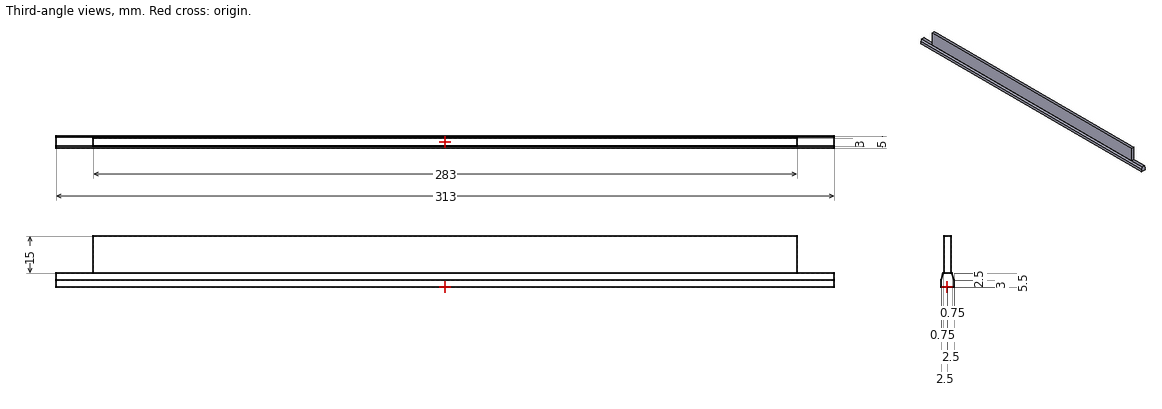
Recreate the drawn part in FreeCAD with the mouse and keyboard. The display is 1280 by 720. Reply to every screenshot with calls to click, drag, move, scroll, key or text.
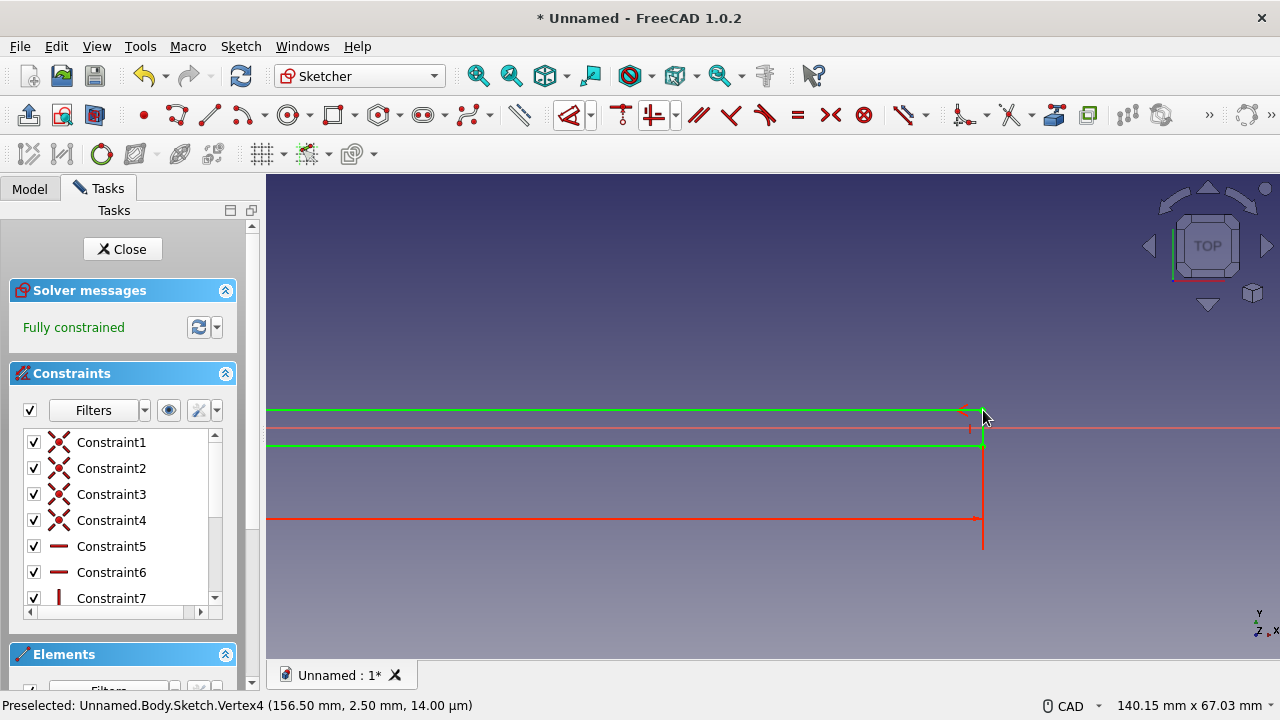
click(123, 249)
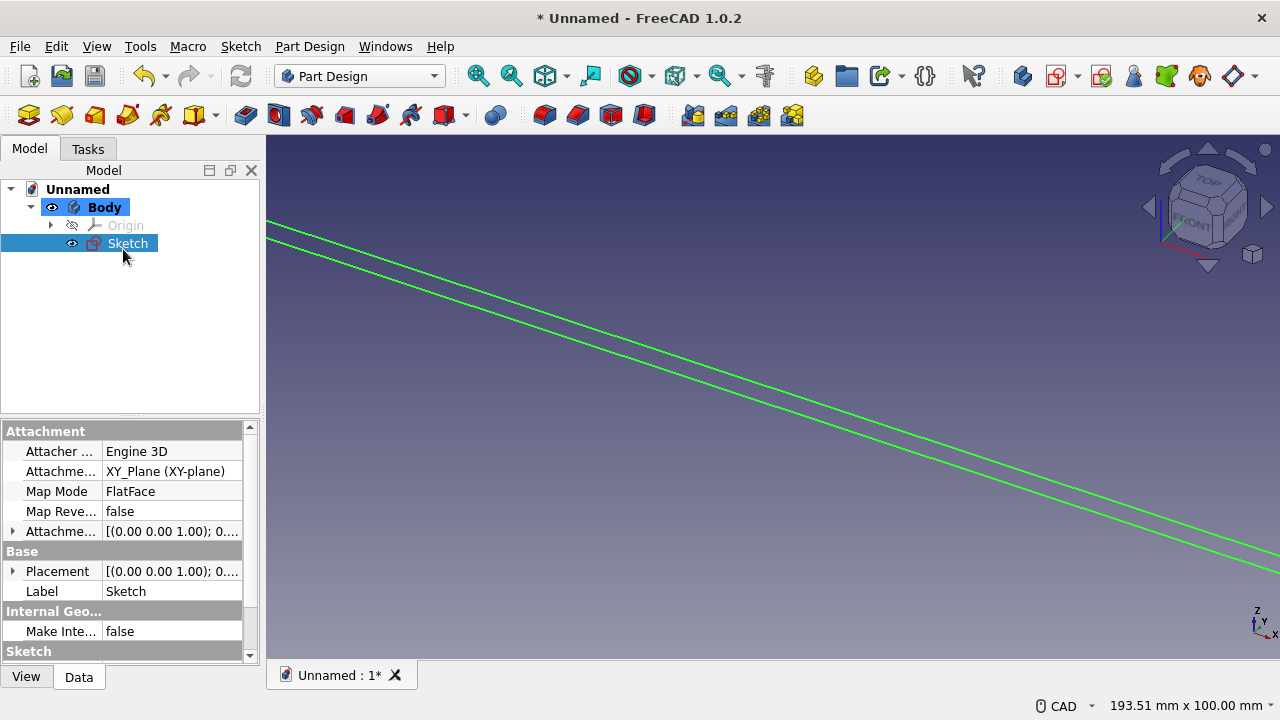
click(29, 116)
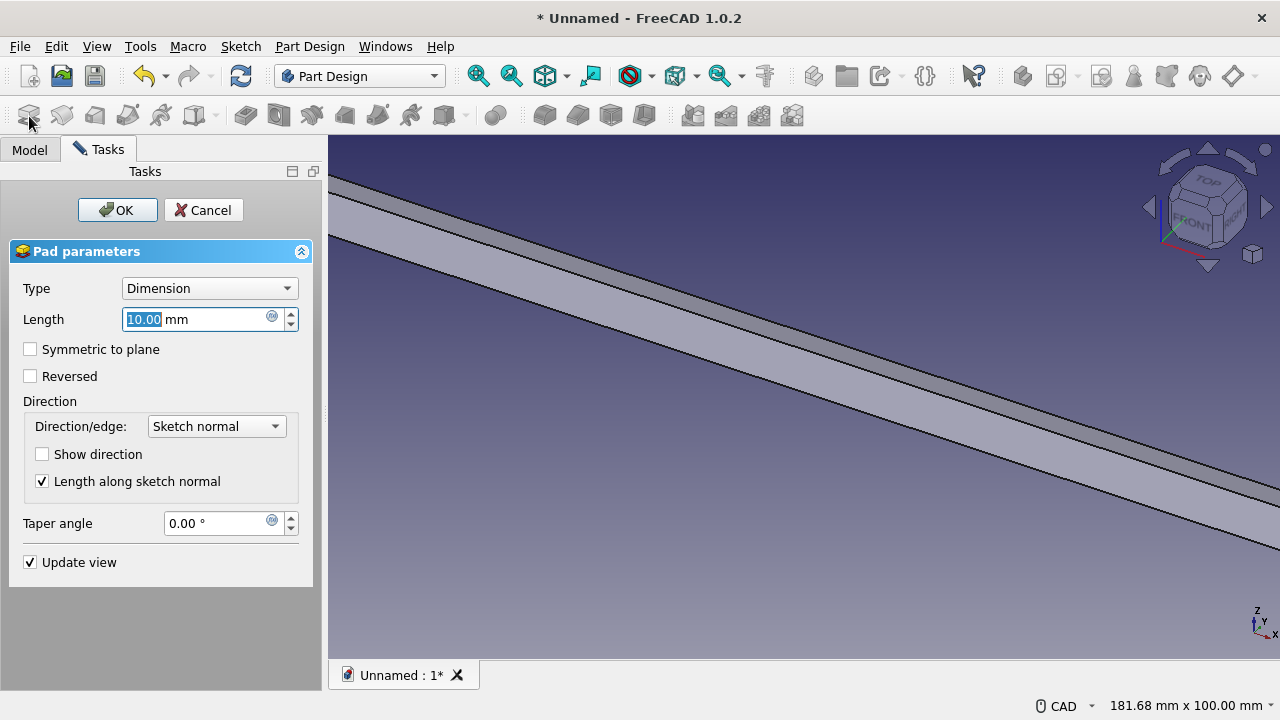
text(5.5)
key(Tab)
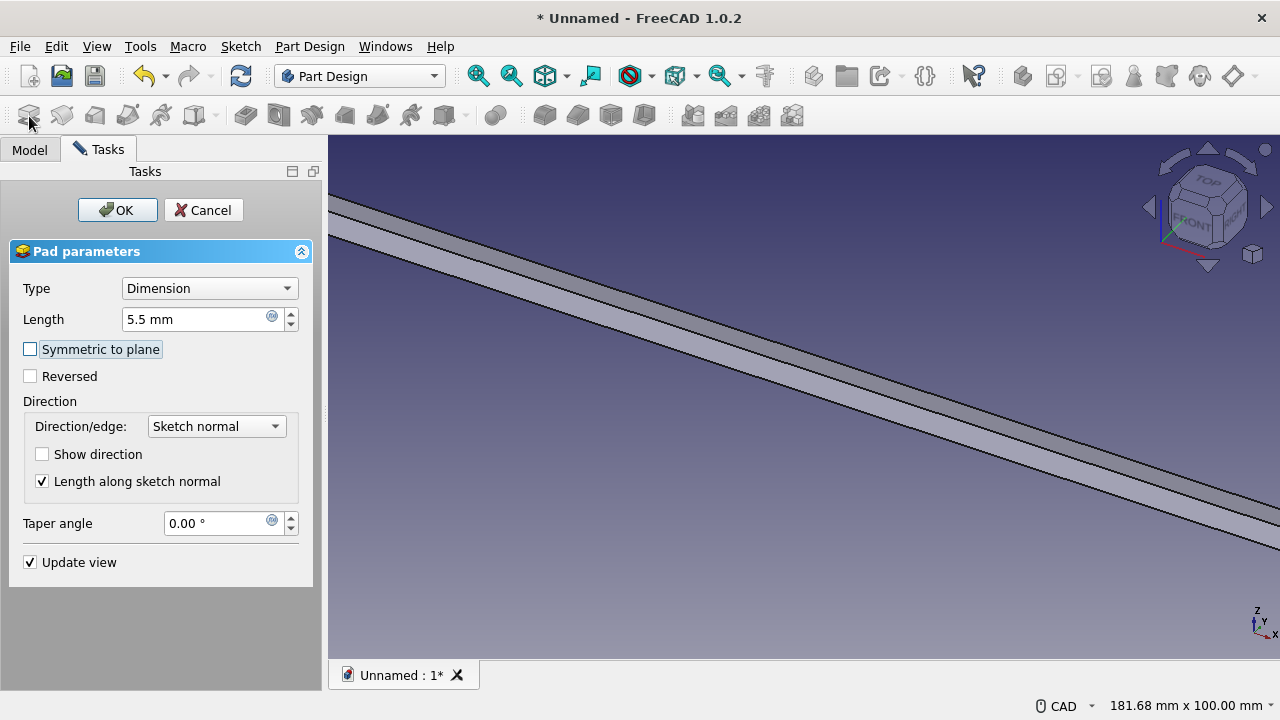
click(118, 210)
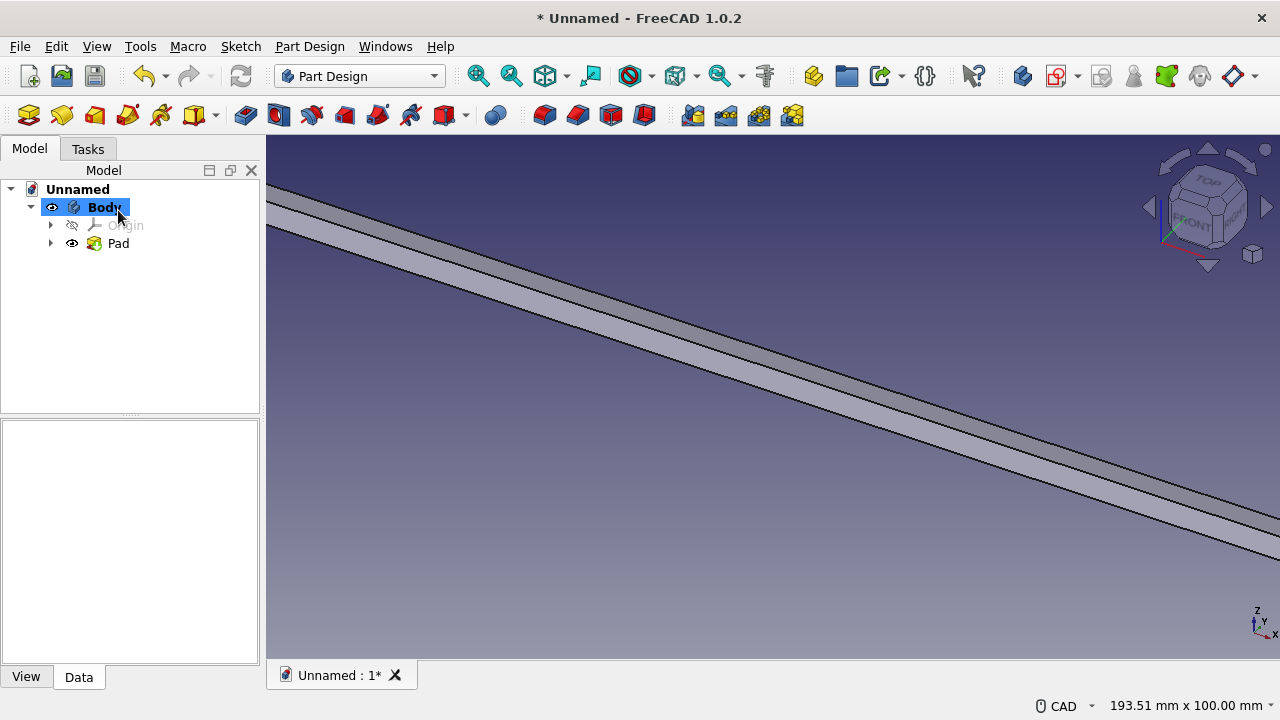
click(479, 76)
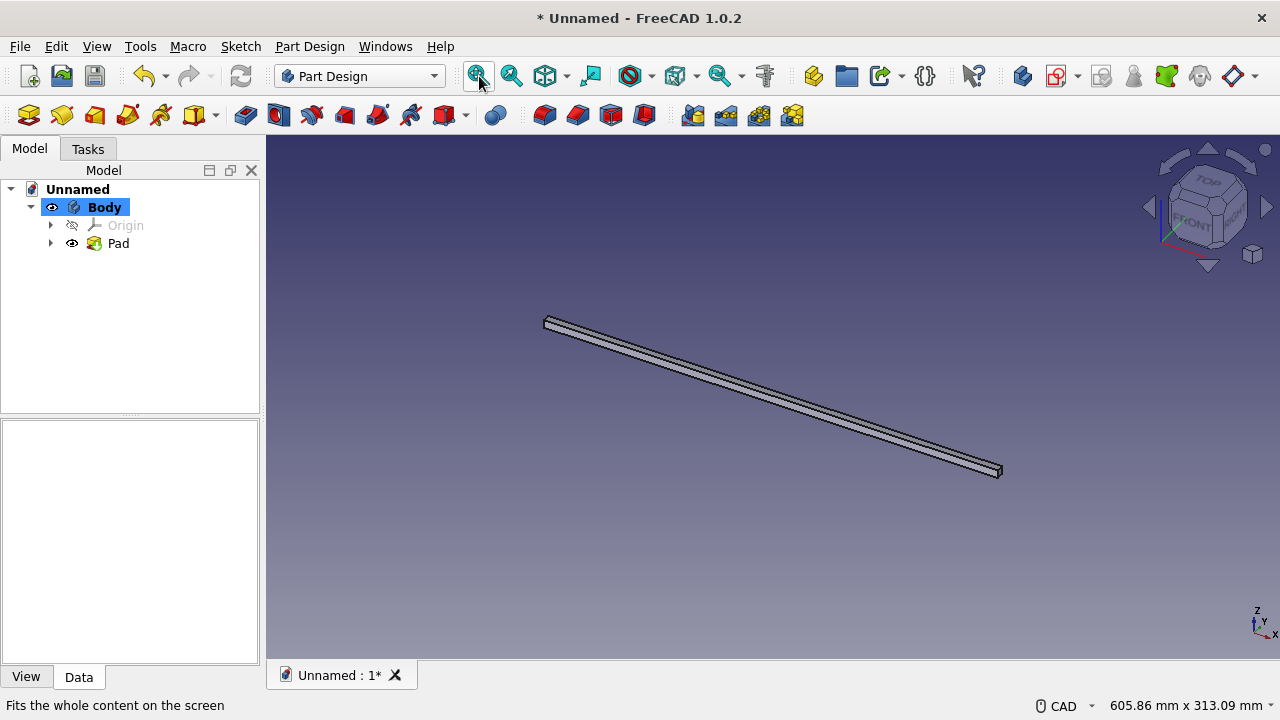
scroll(1000, 471, up, 6)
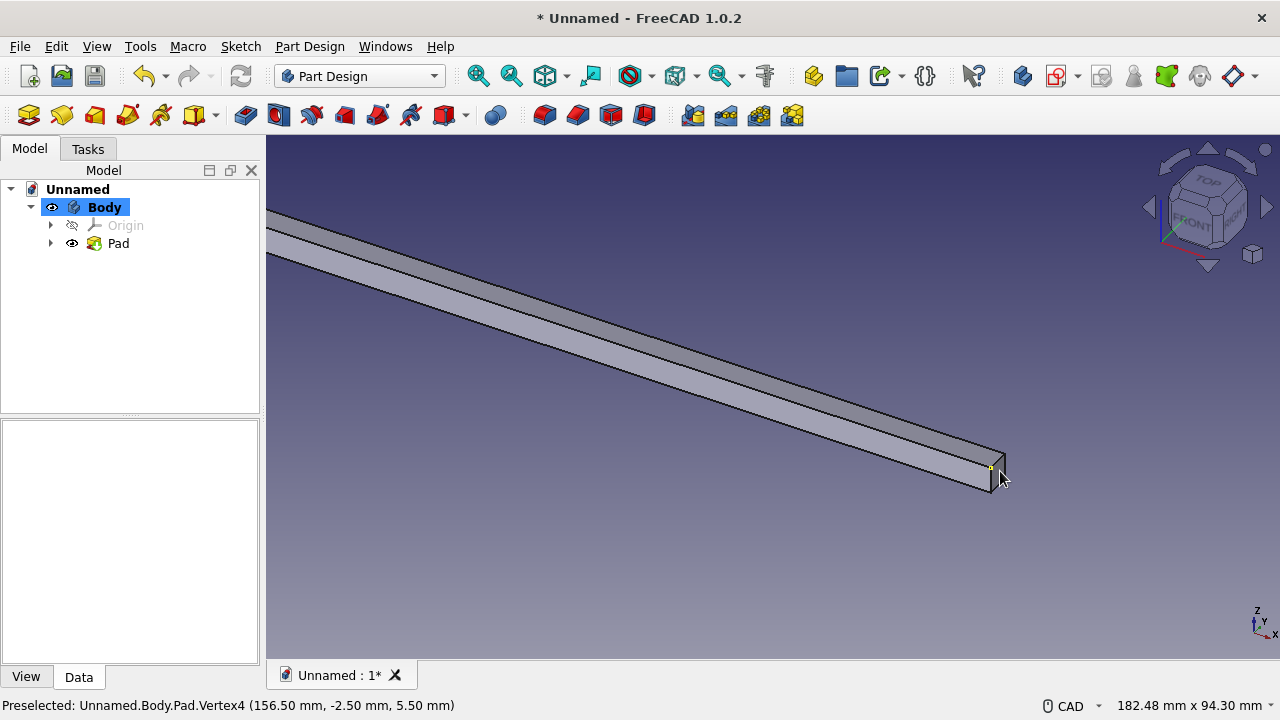
click(479, 76)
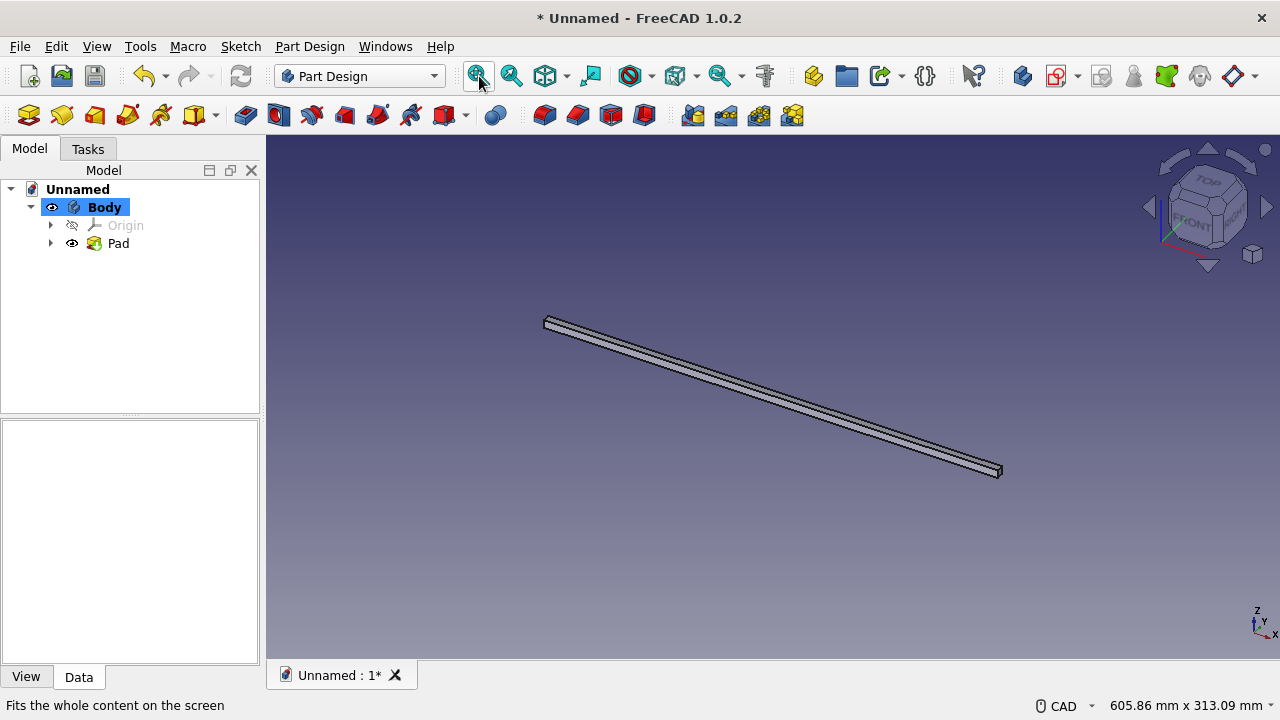
key(0)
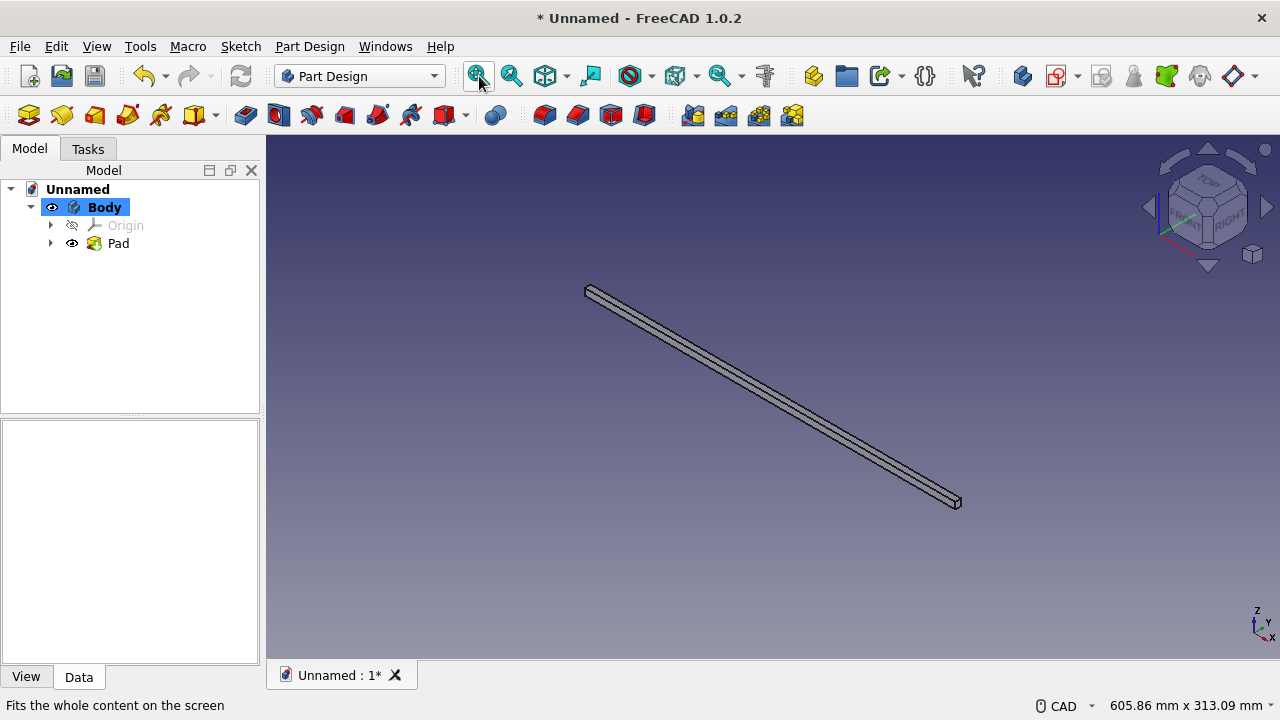
click(479, 76)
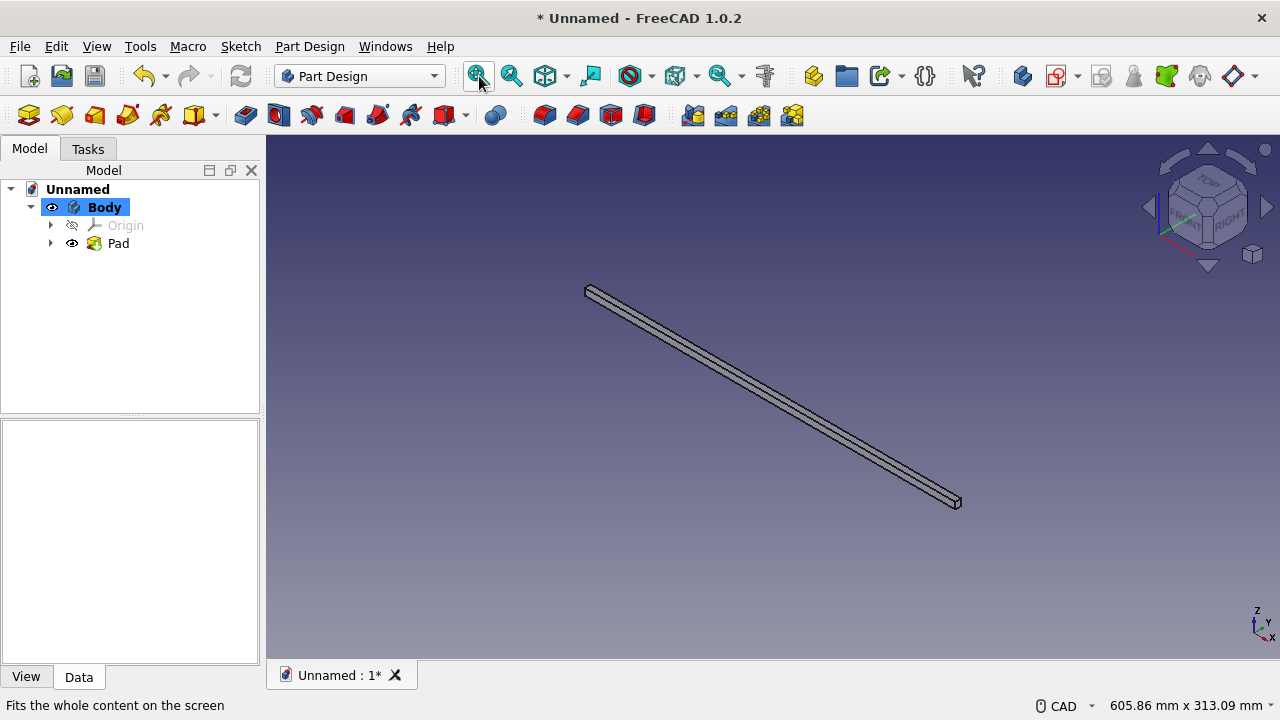
scroll(958, 503, up, 6)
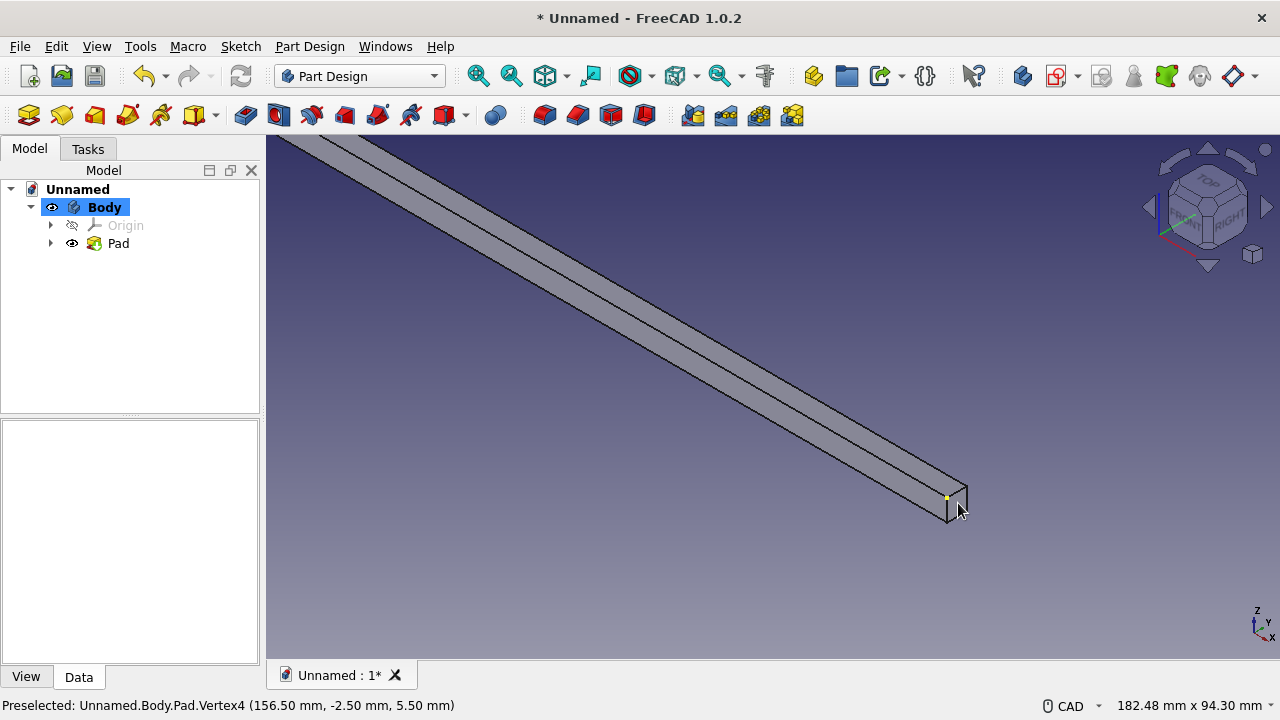
click(957, 503)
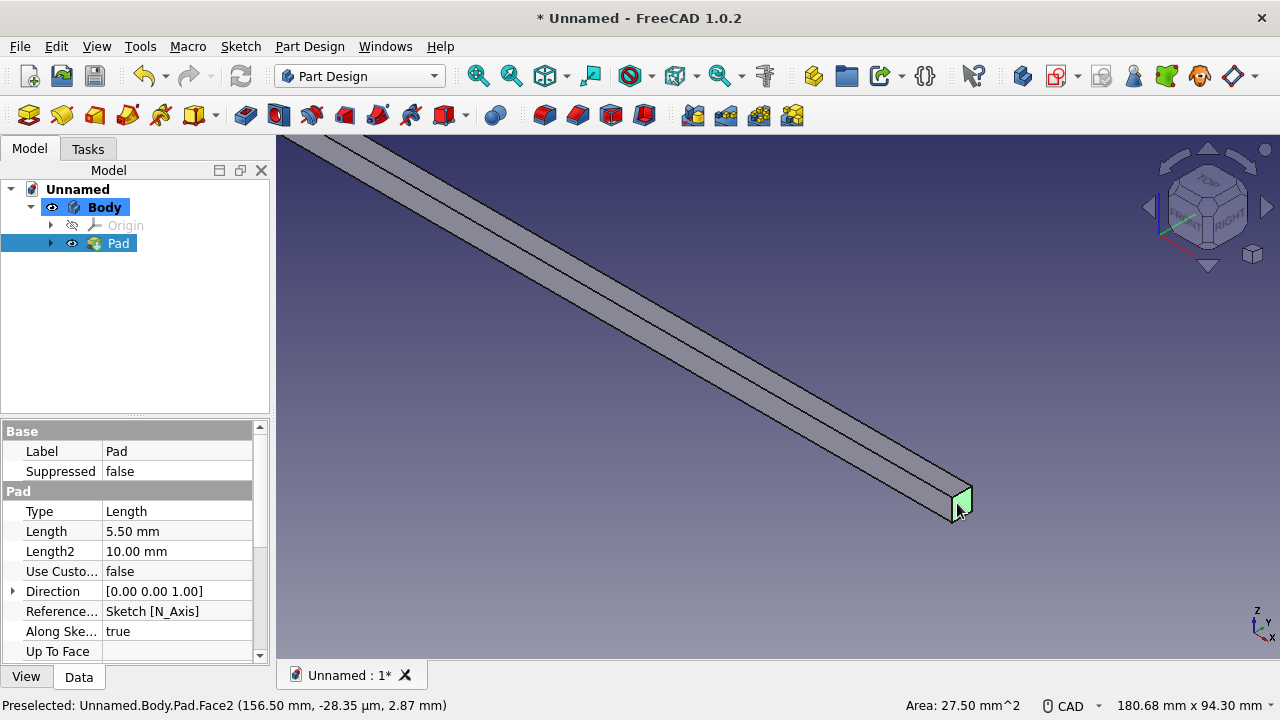
click(1056, 76)